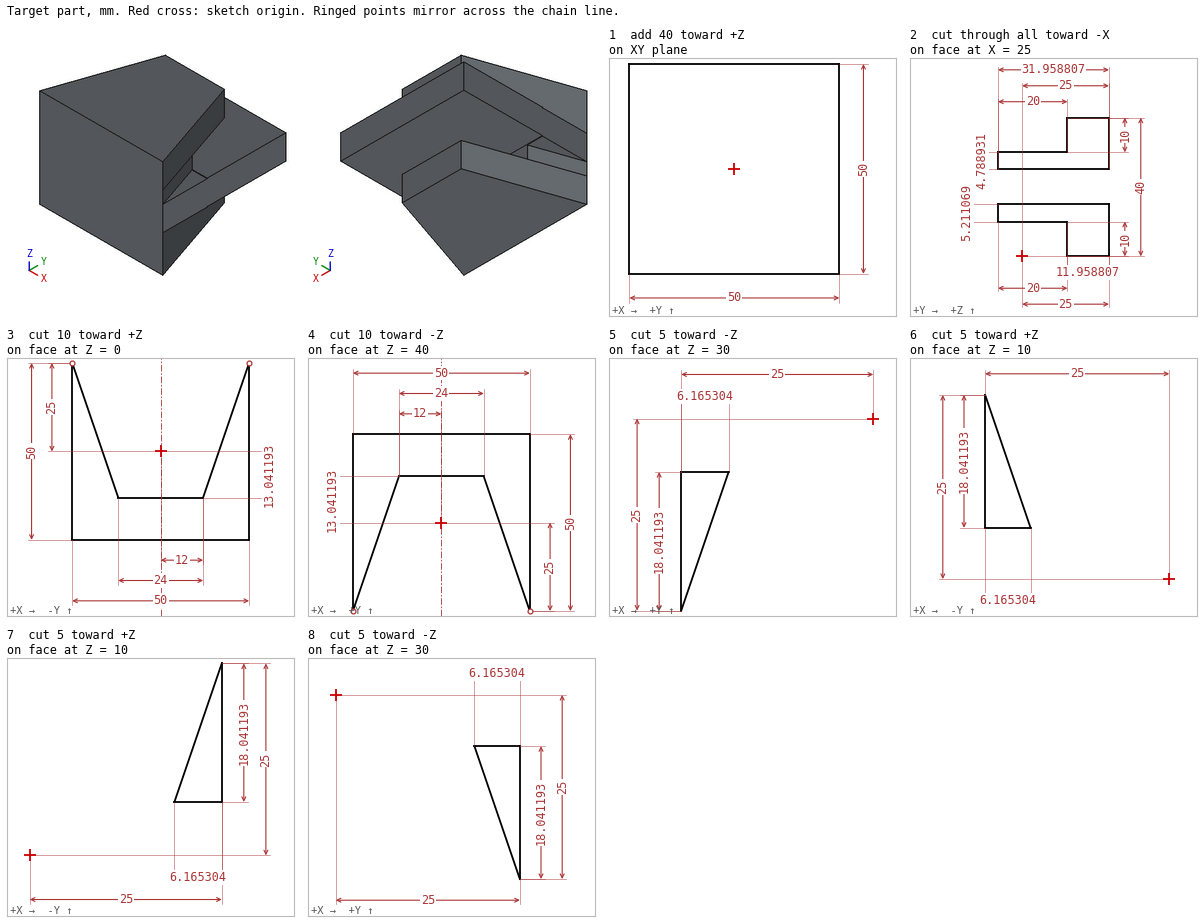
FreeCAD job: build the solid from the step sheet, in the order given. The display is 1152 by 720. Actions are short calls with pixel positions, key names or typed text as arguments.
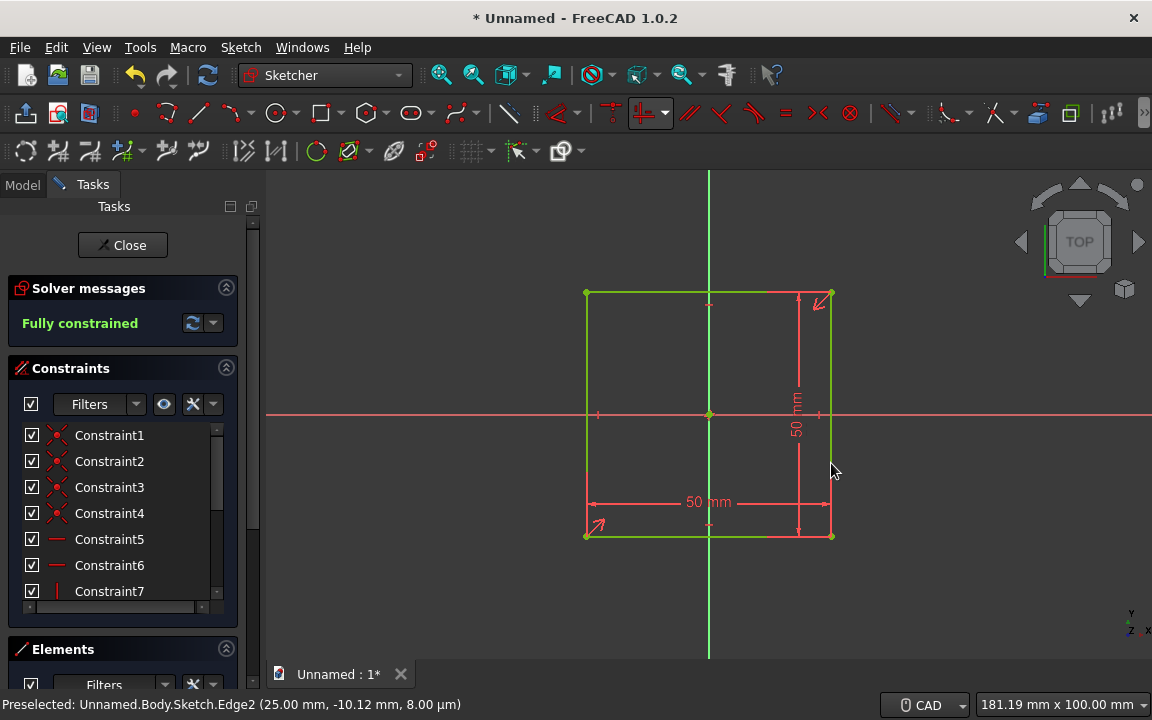
click(123, 245)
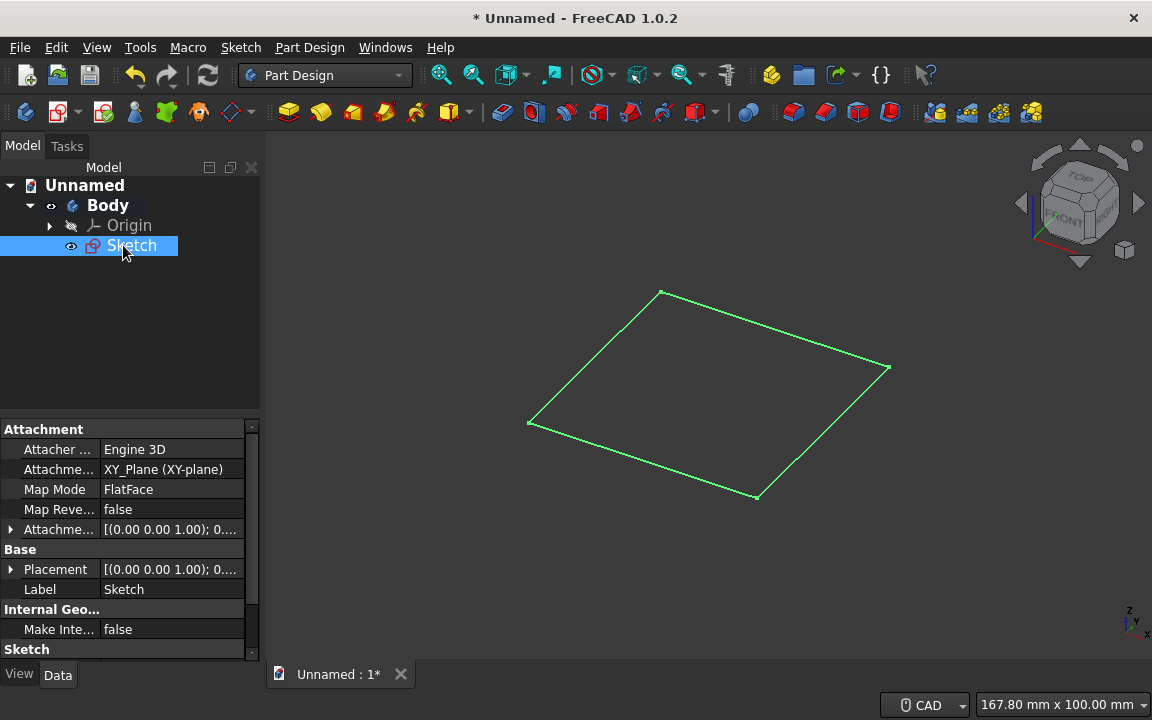
click(290, 112)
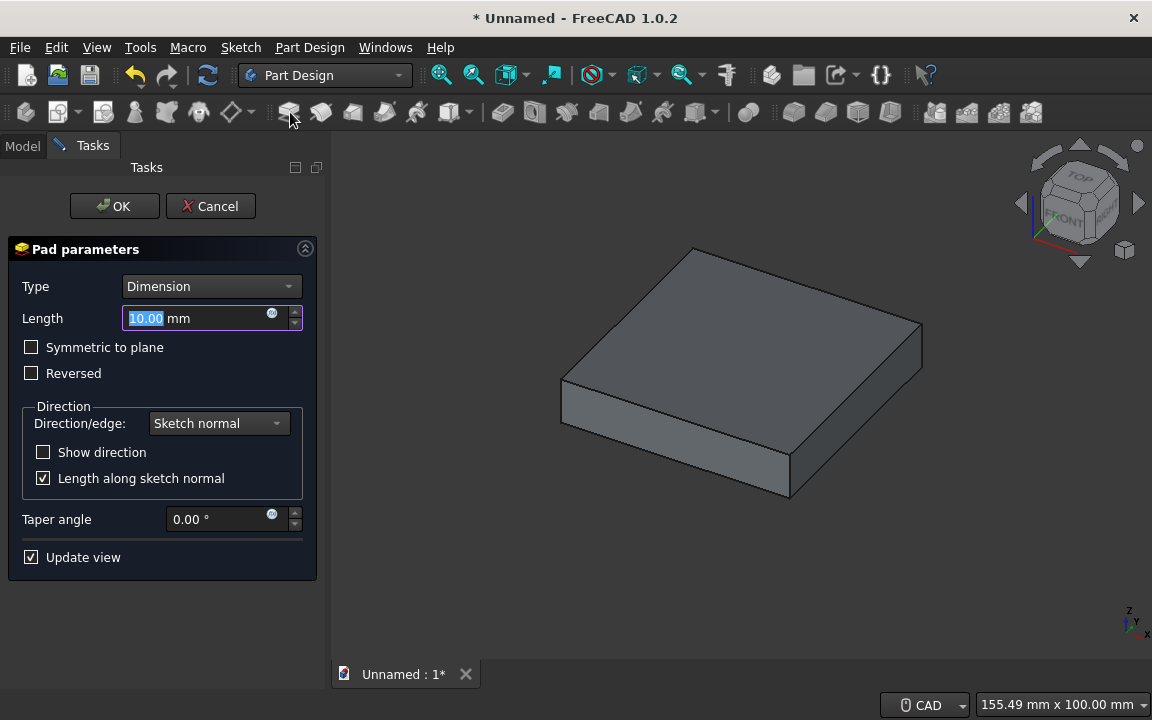
text(40)
key(Tab)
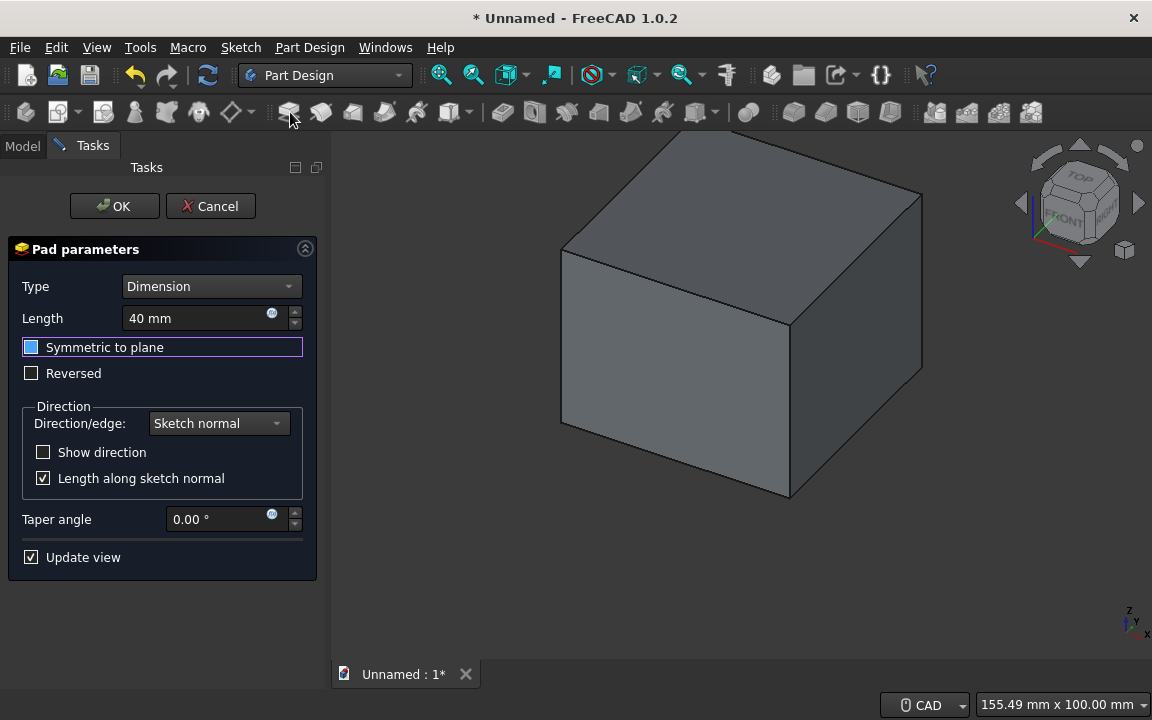
click(115, 206)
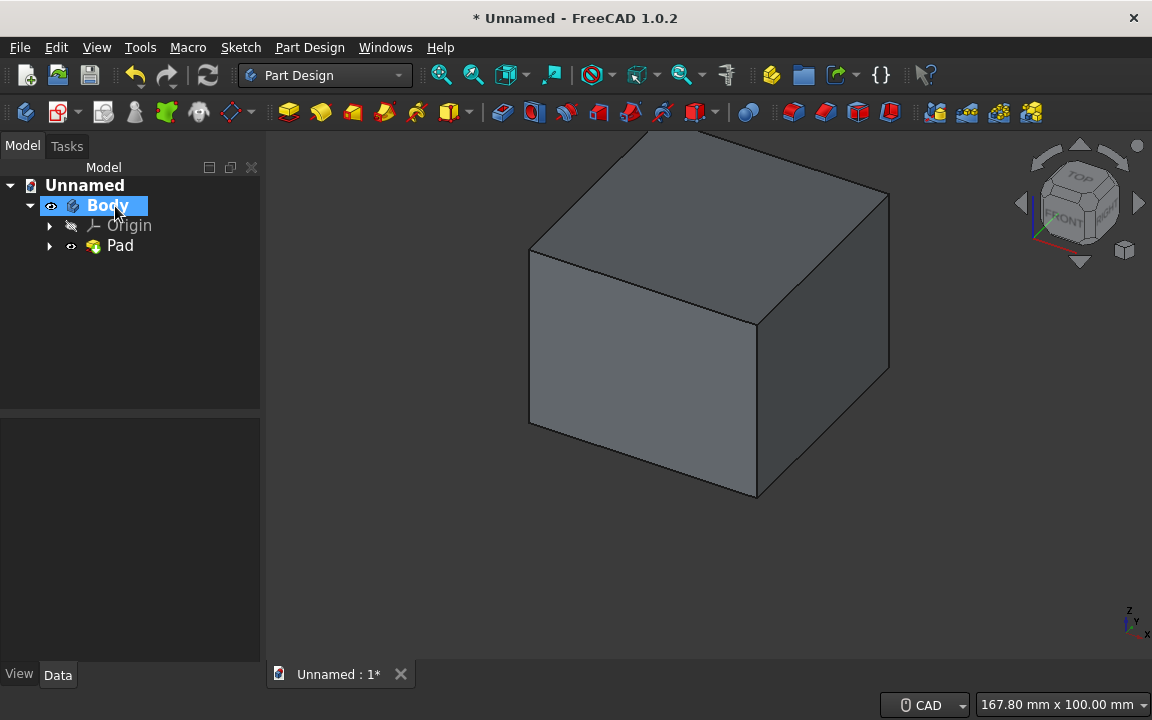
click(442, 76)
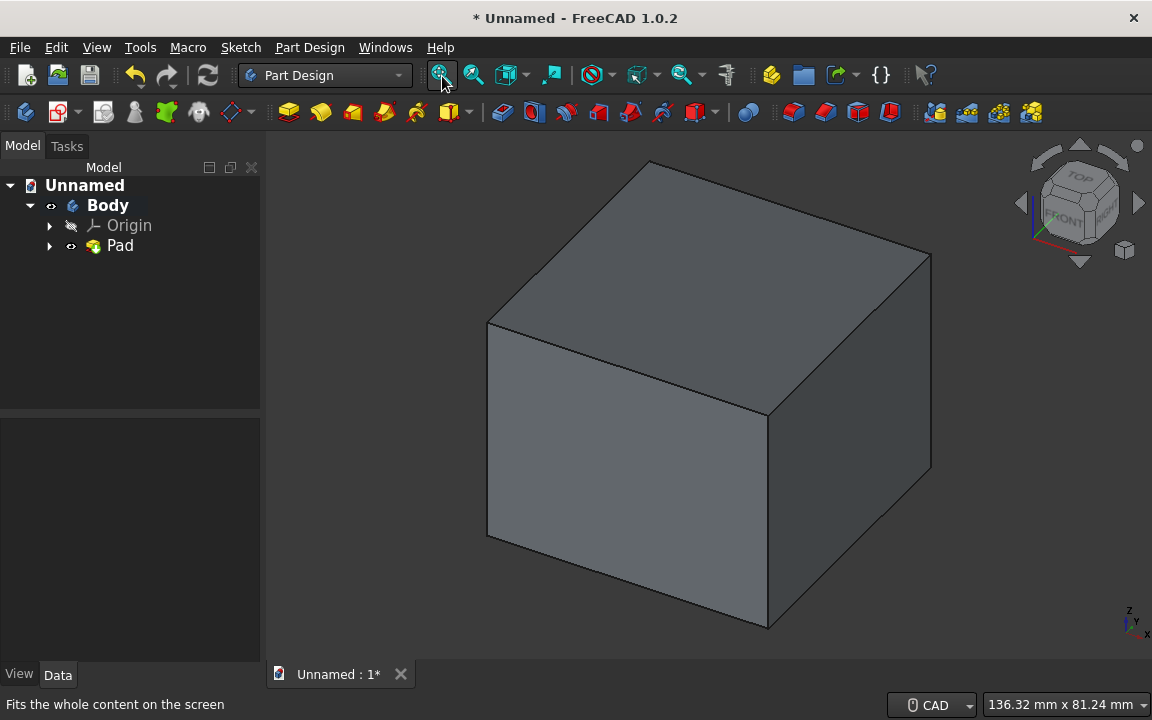
click(850, 441)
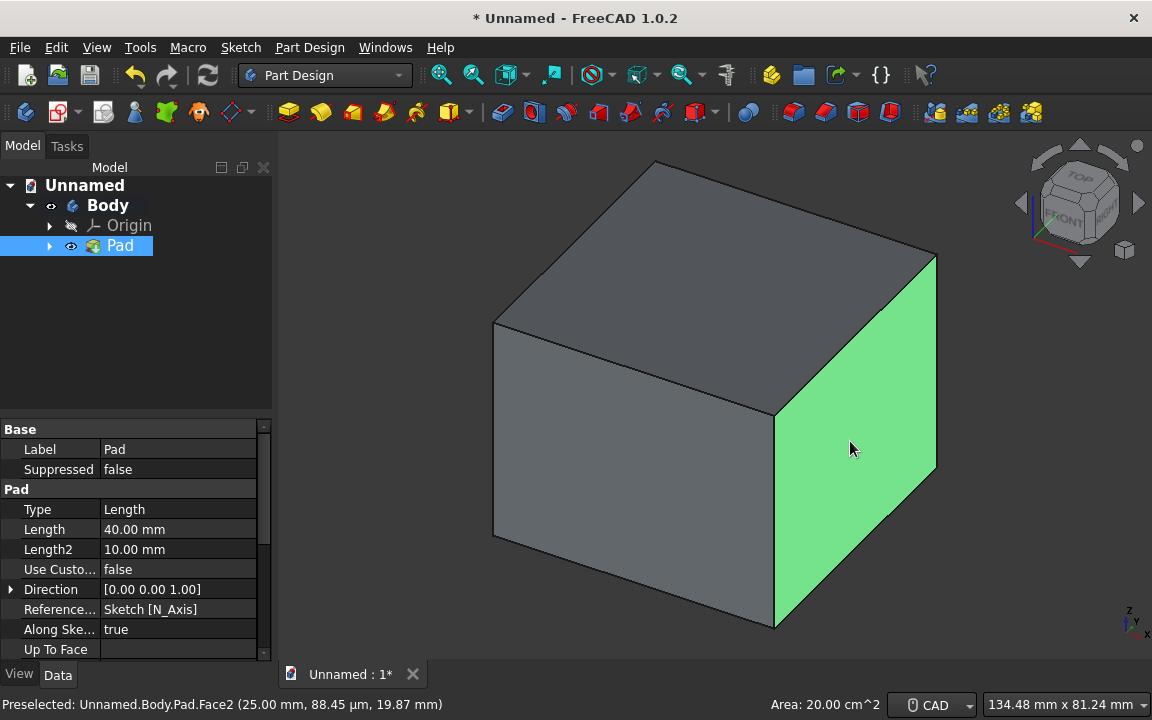
click(58, 112)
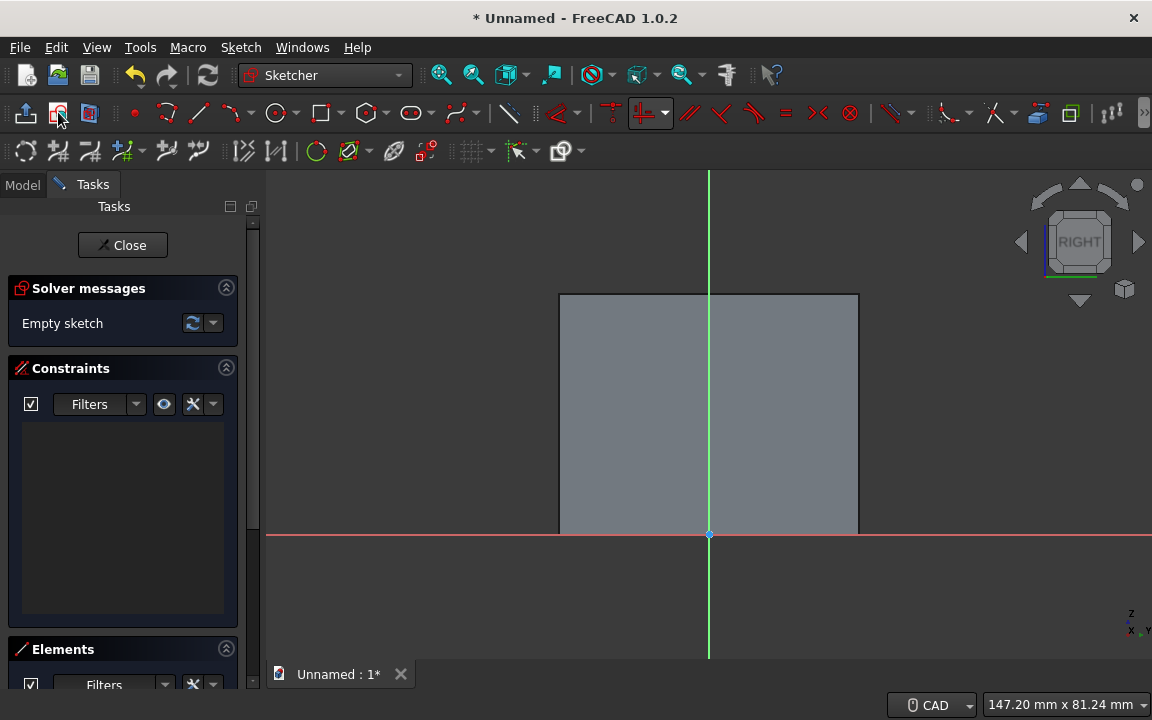
key(g)
key(m)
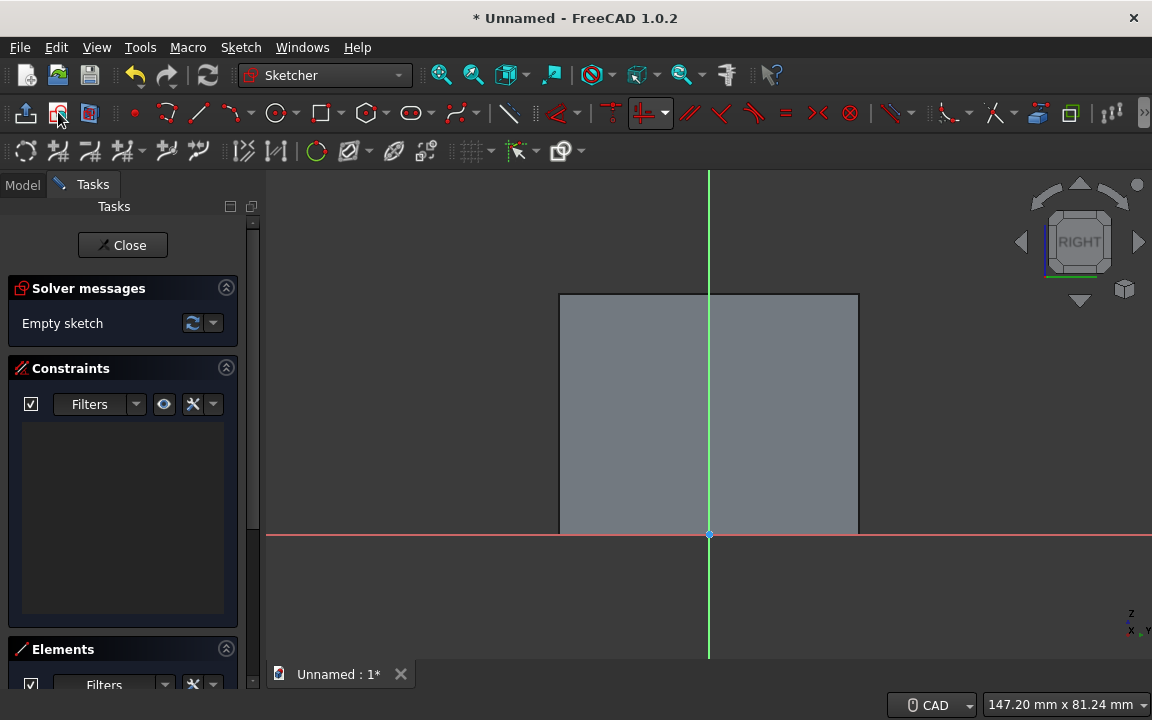
click(667, 383)
click(859, 383)
click(859, 294)
click(787, 294)
click(787, 354)
click(667, 354)
click(667, 384)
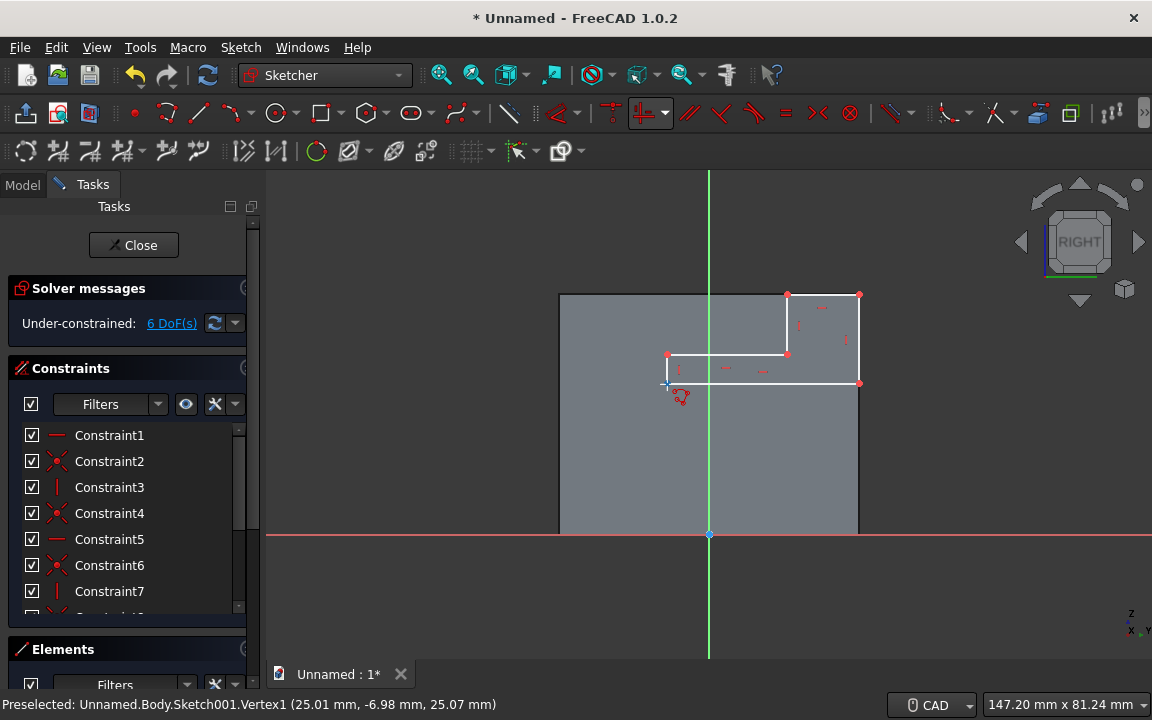
click(667, 475)
click(787, 475)
click(787, 535)
click(859, 526)
click(859, 443)
click(667, 443)
click(667, 476)
key(Escape)
key(Escape)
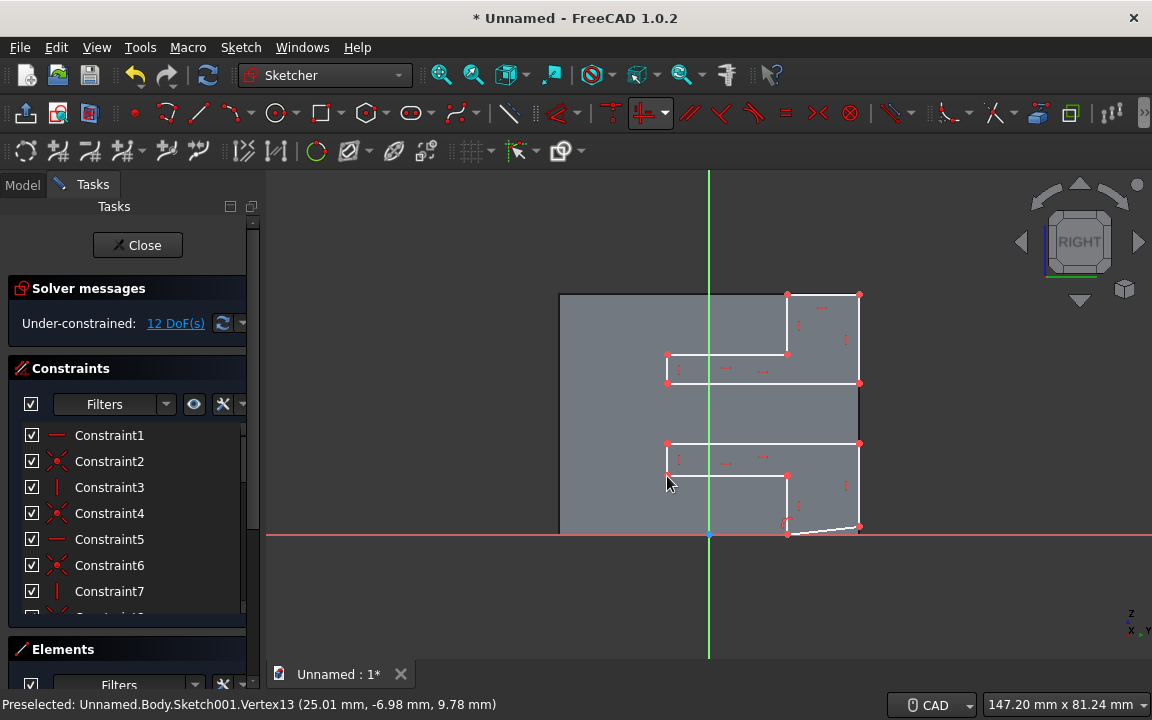
click(809, 533)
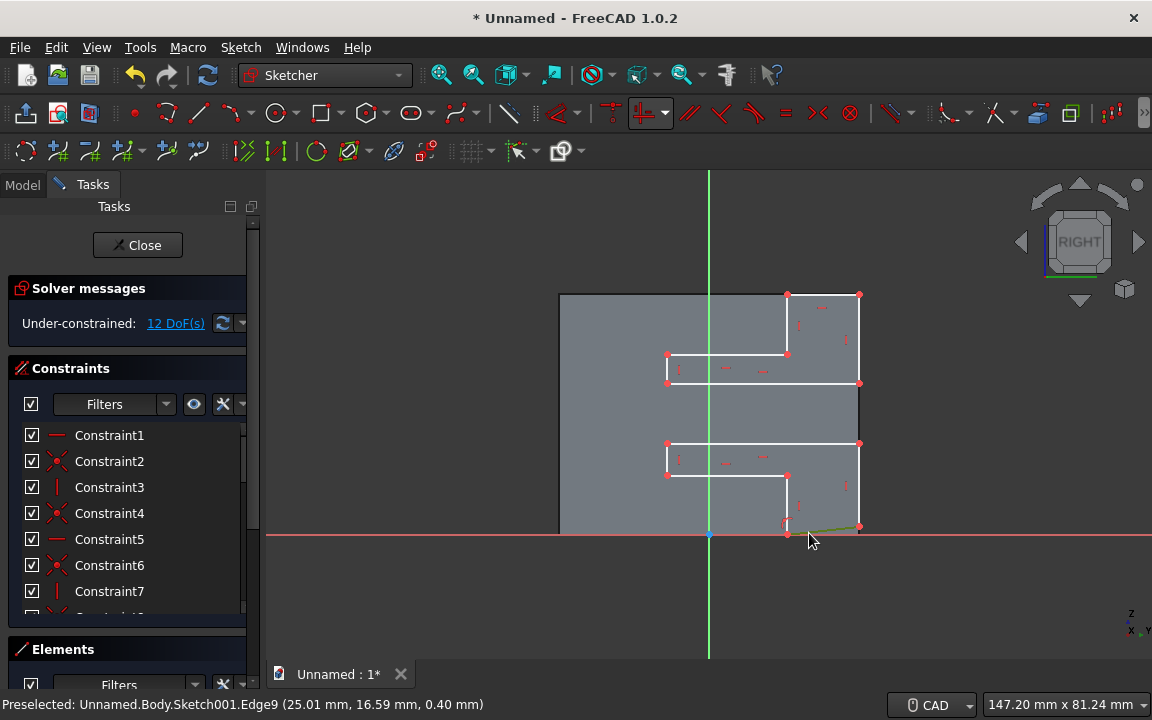
click(668, 114)